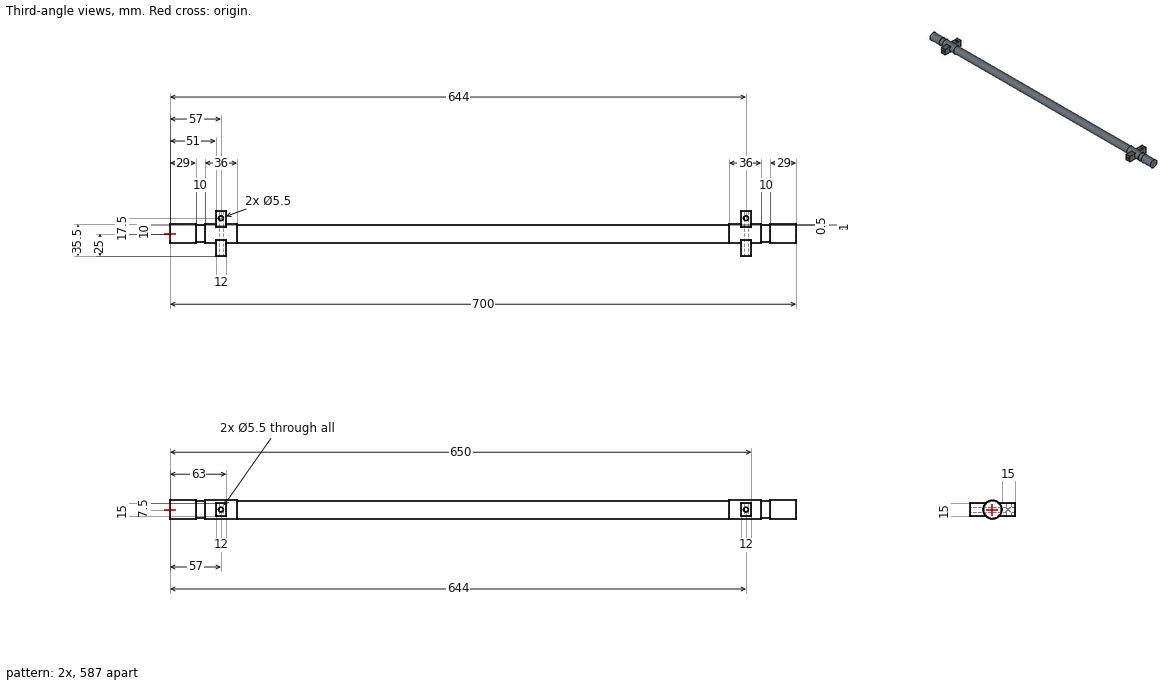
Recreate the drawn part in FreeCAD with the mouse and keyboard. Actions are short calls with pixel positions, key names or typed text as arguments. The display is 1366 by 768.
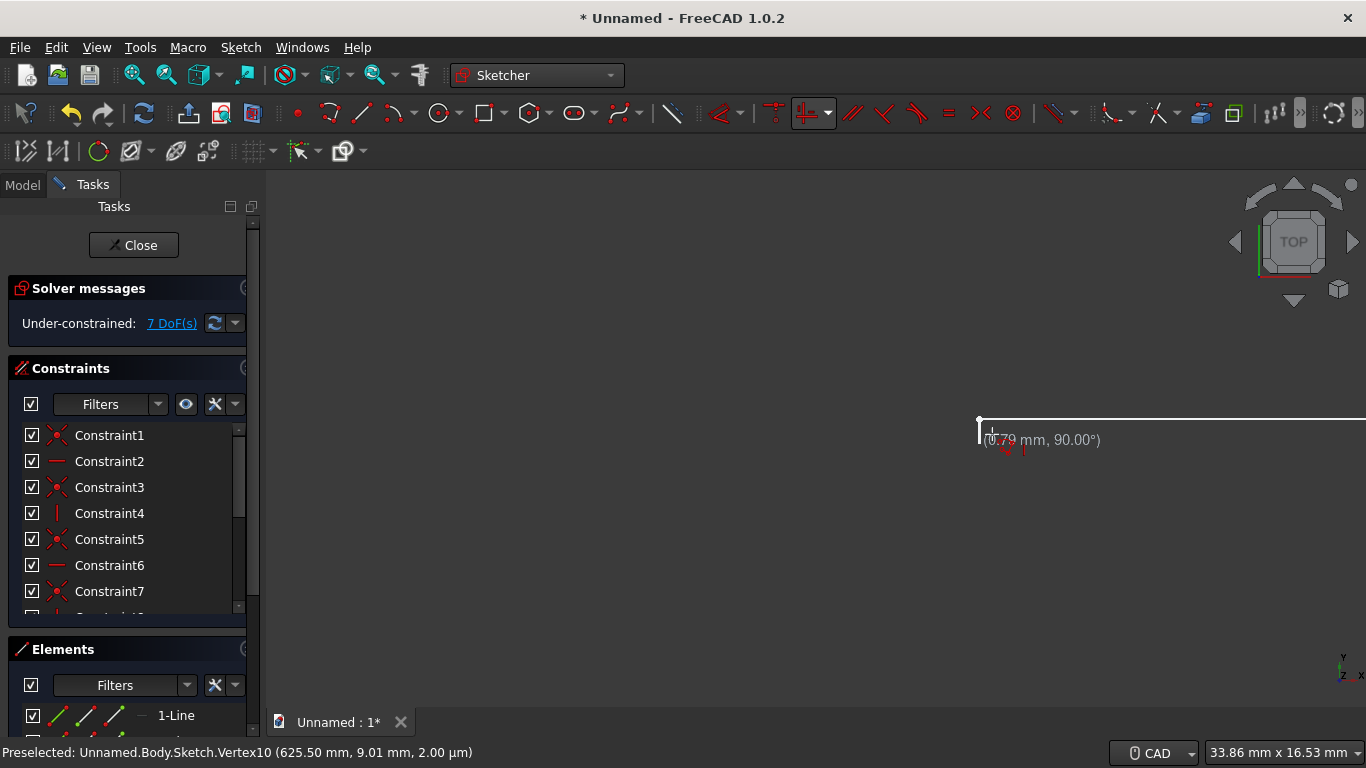
click(979, 433)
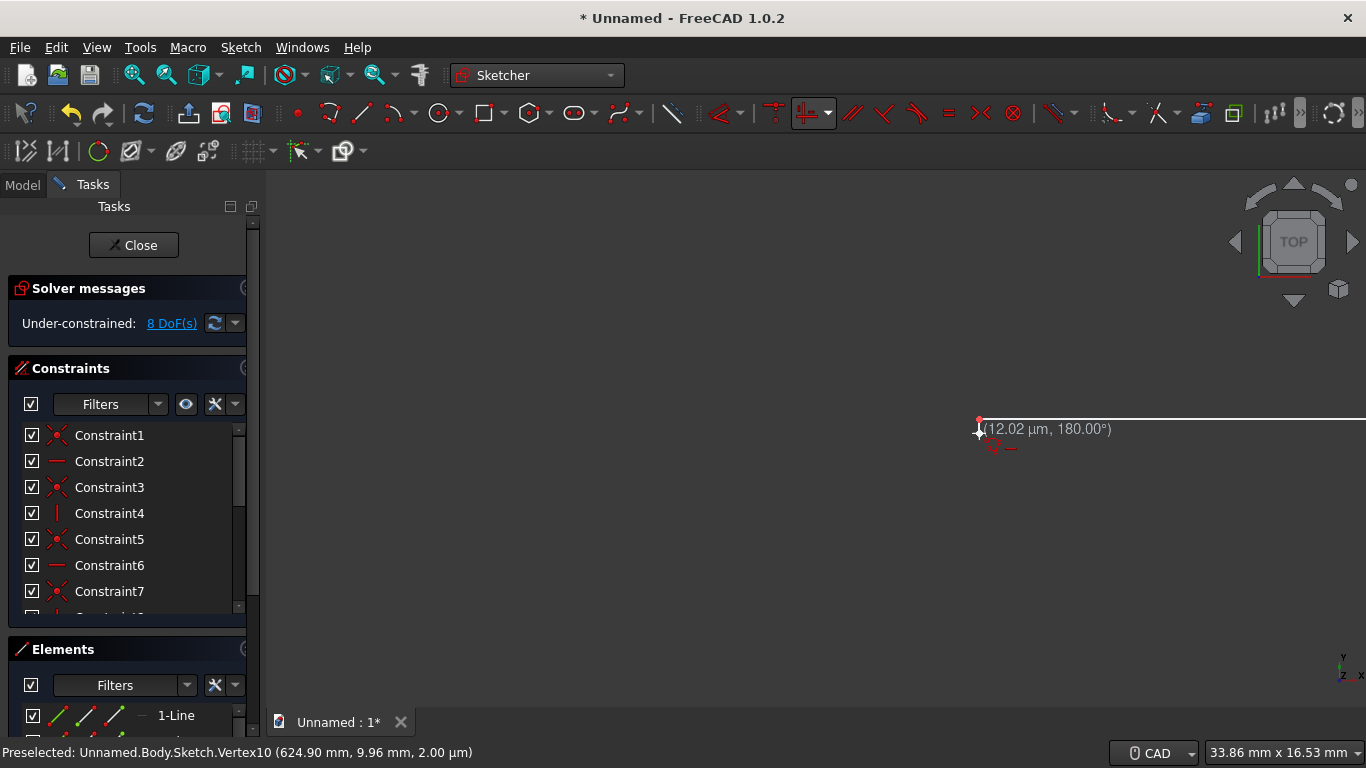
scroll(1048, 433, down, 17)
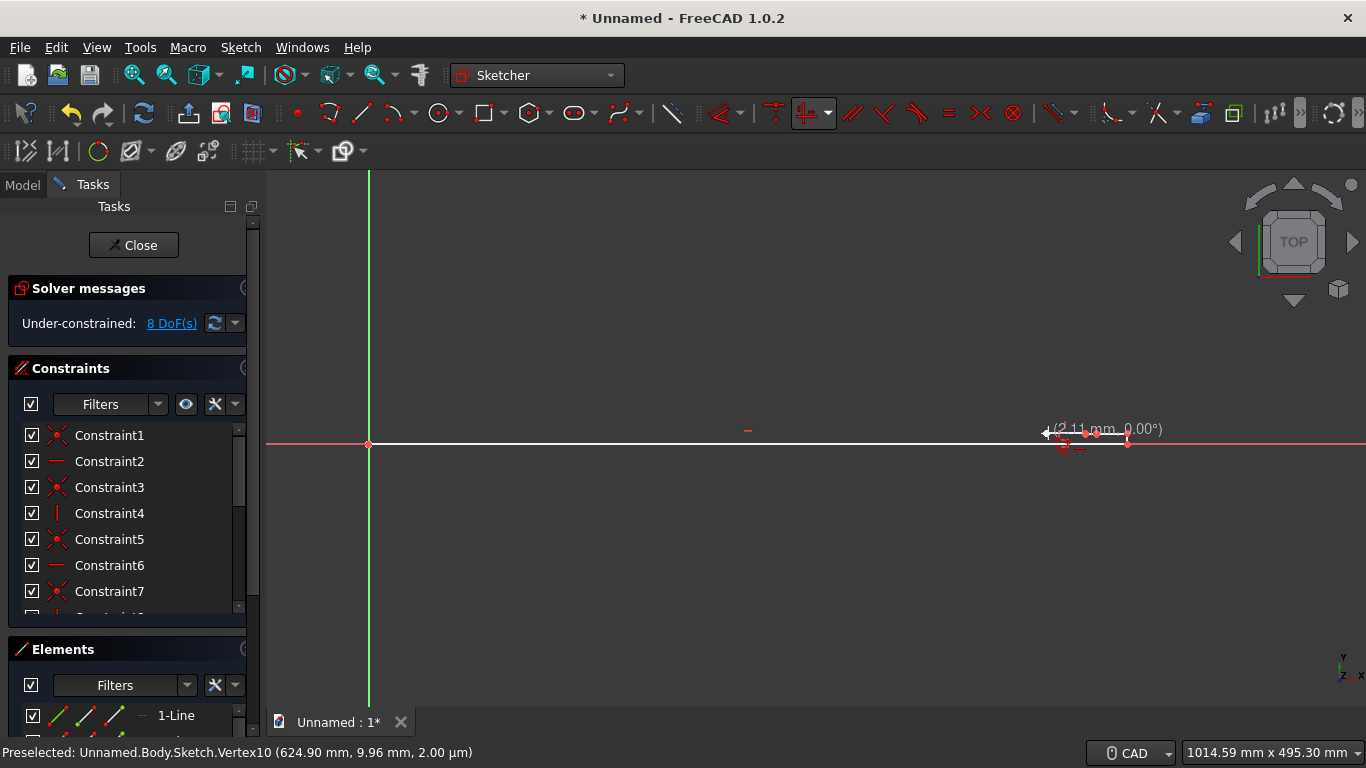
scroll(450, 433, up, 2)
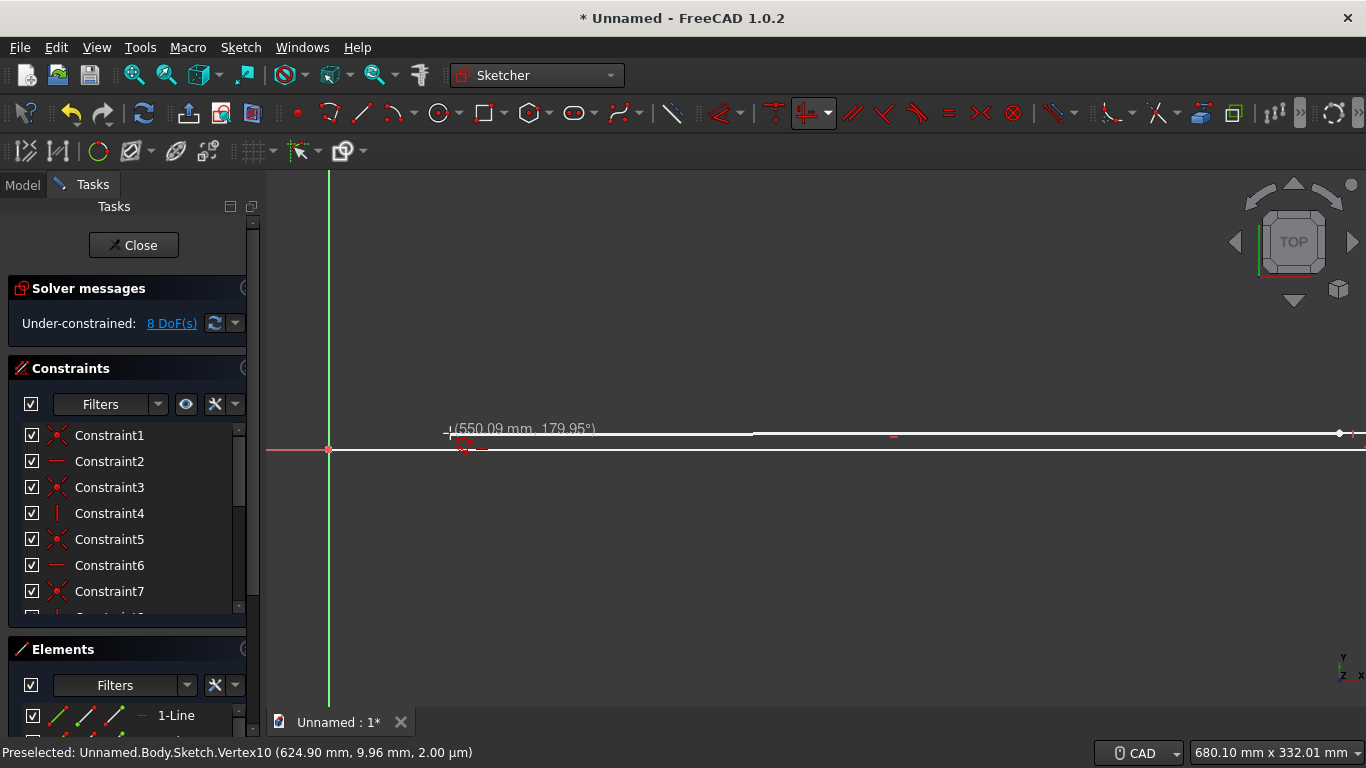
click(450, 433)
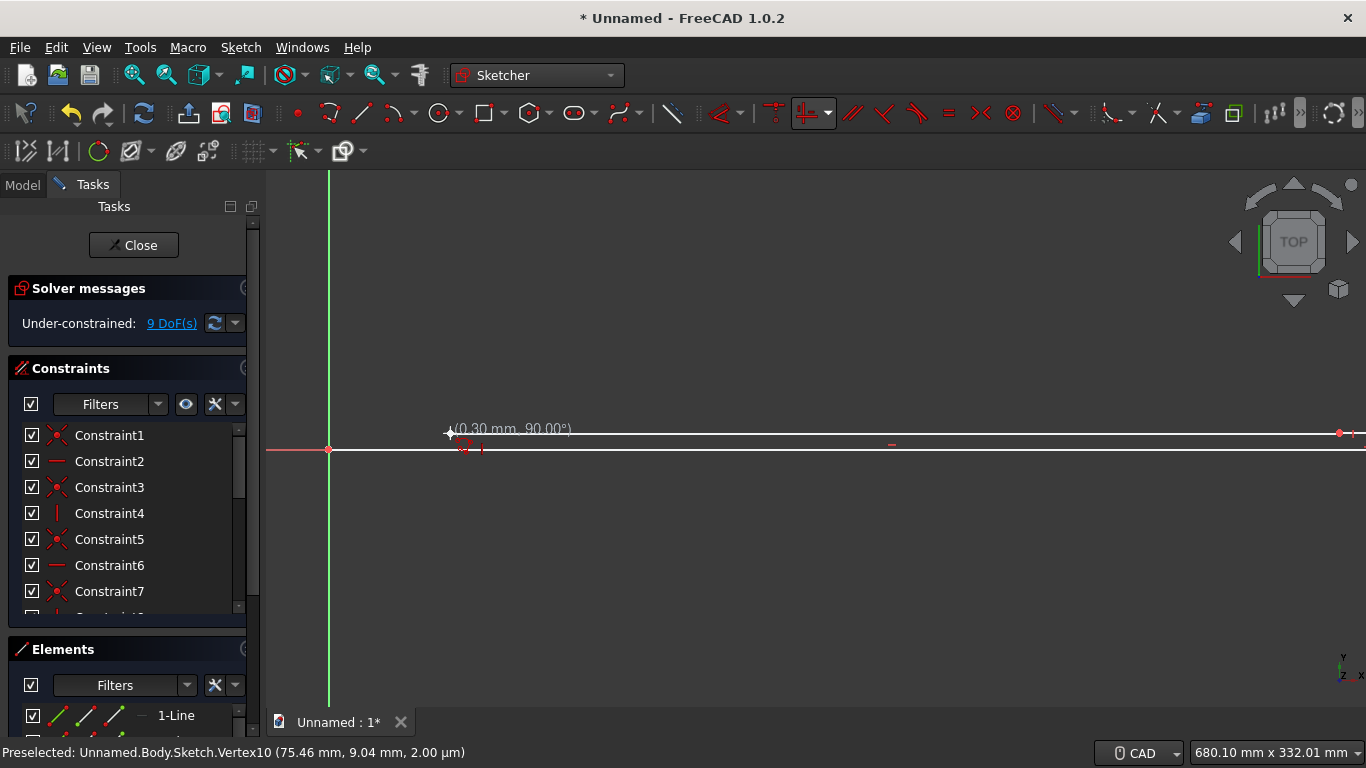
scroll(450, 433, up, 15)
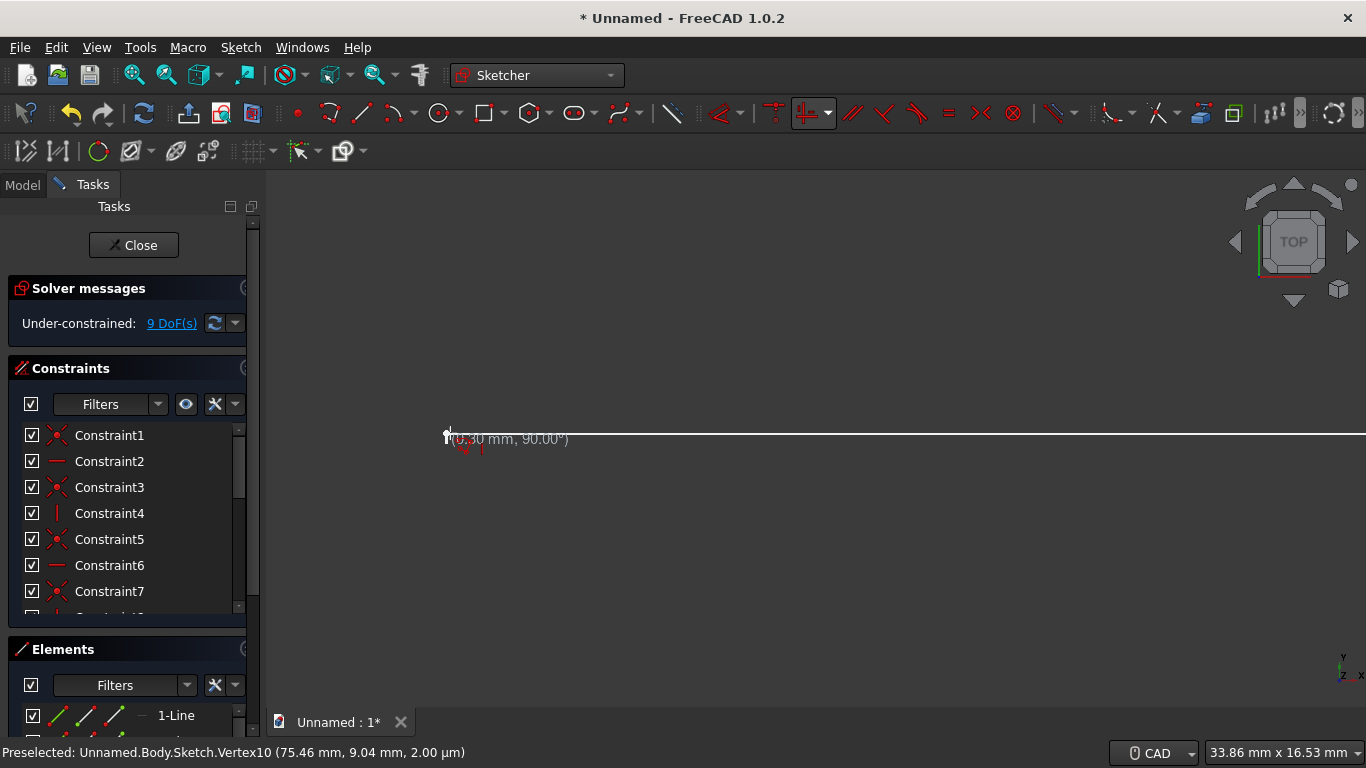
click(447, 416)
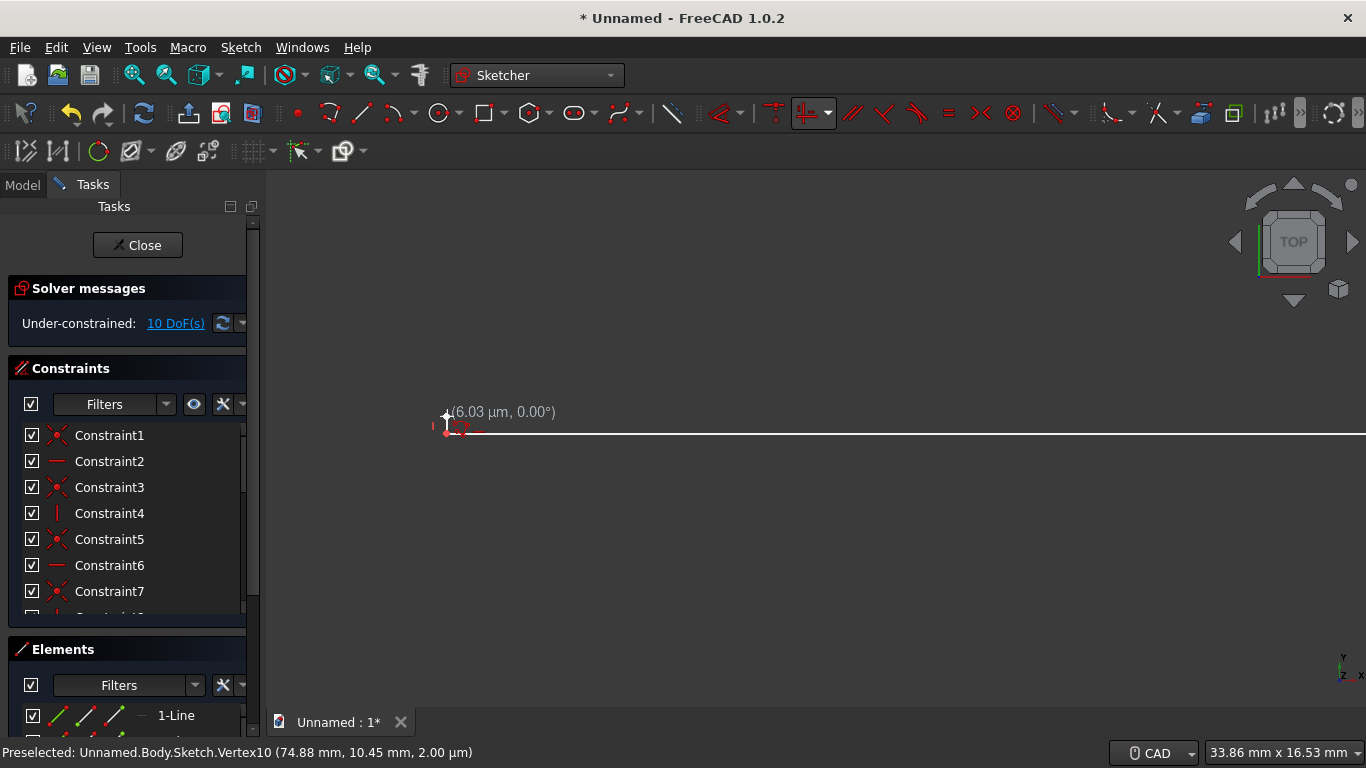
scroll(449, 433, down, 17)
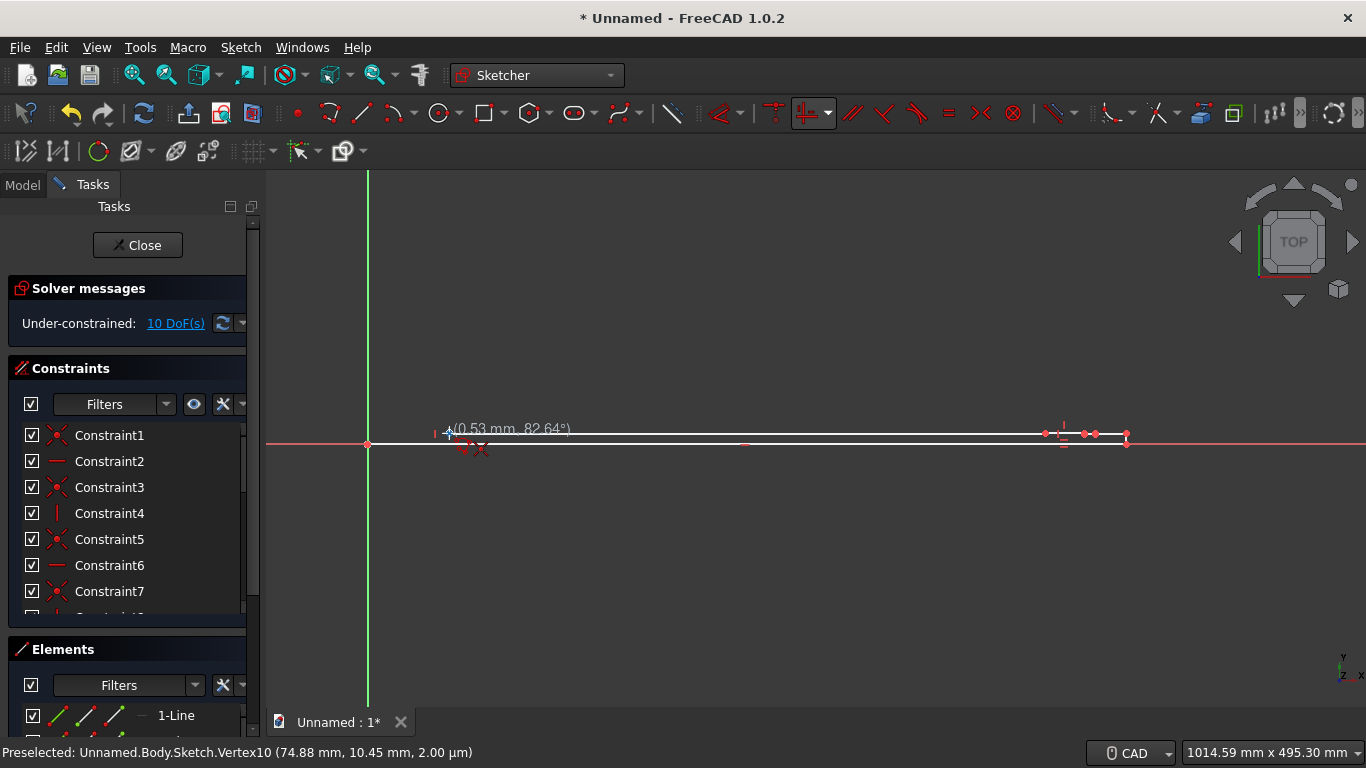
scroll(410, 433, up, 2)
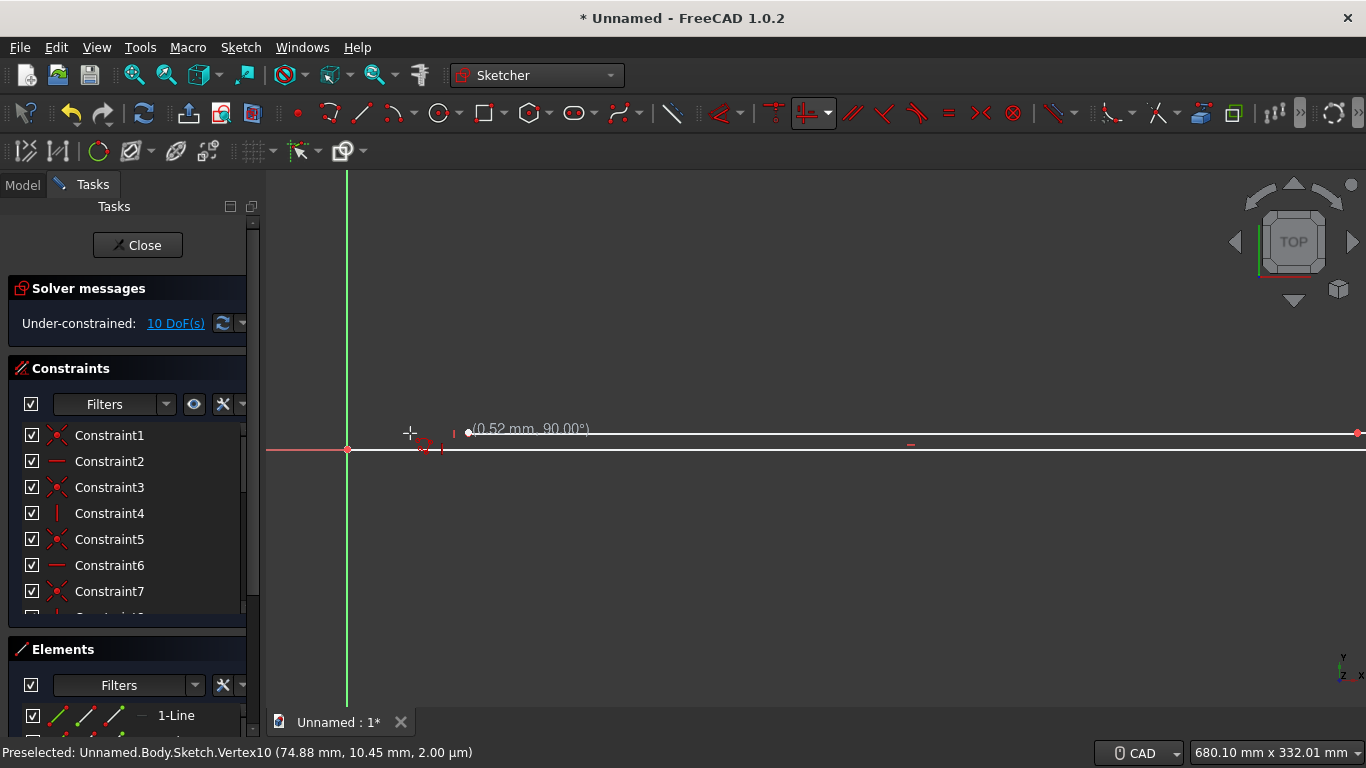
click(410, 433)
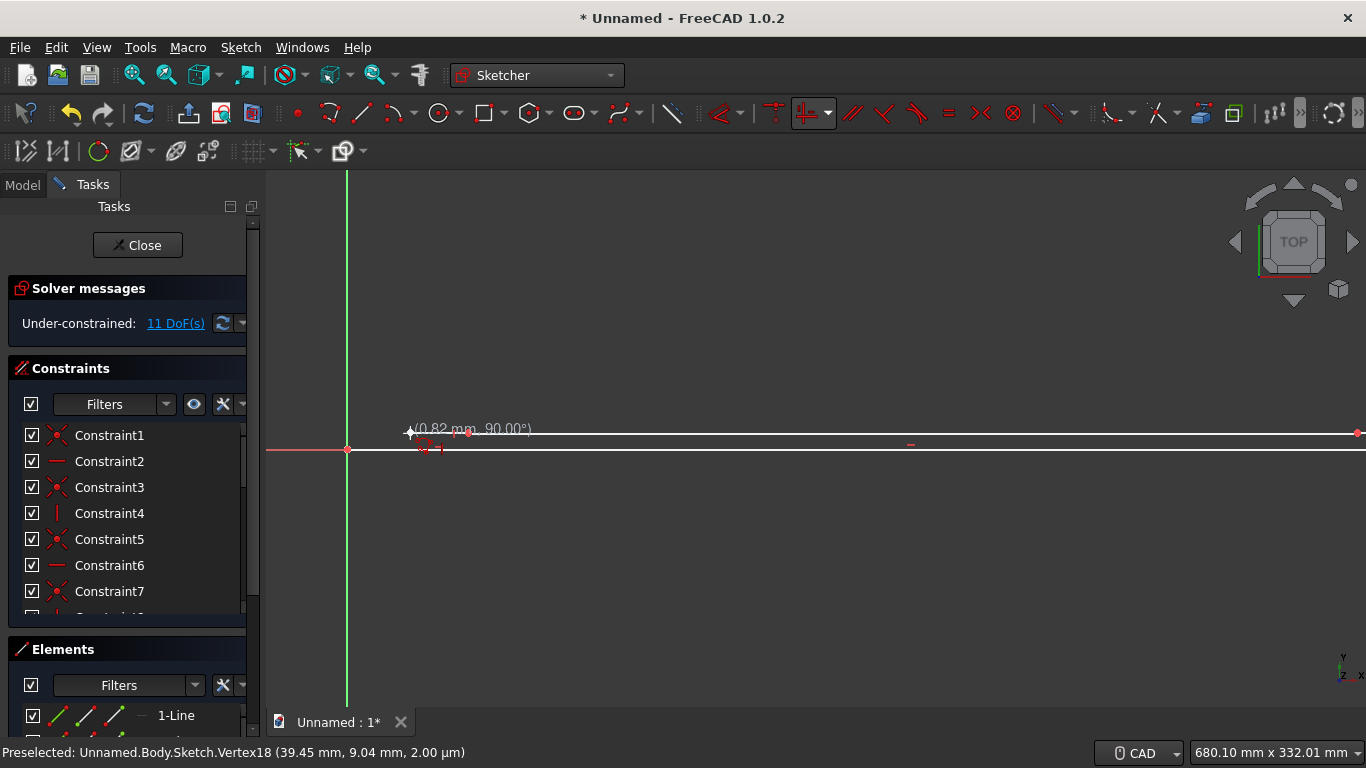
scroll(410, 434, up, 12)